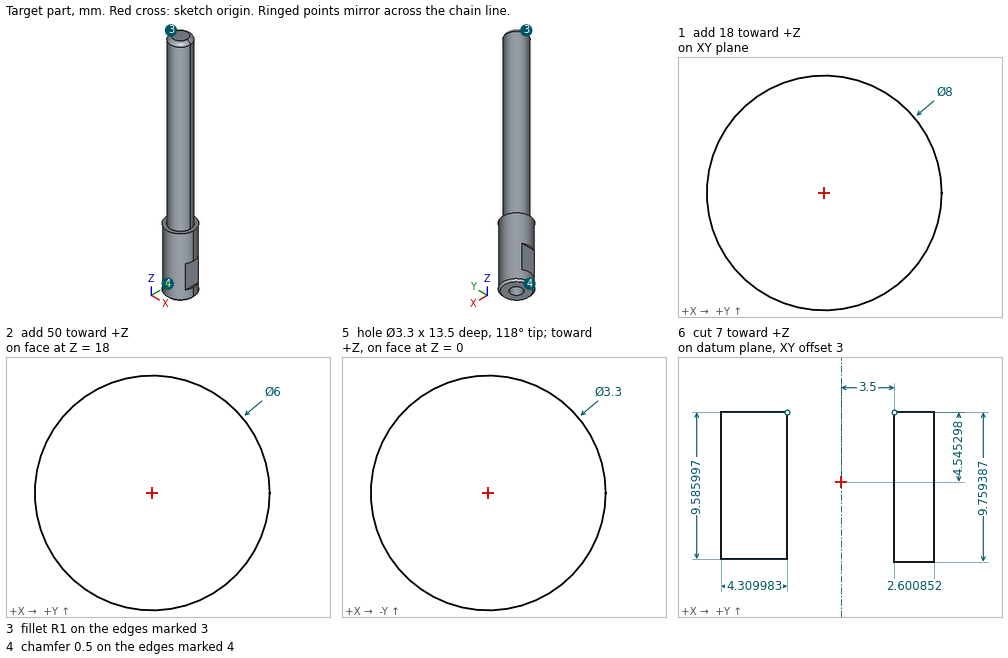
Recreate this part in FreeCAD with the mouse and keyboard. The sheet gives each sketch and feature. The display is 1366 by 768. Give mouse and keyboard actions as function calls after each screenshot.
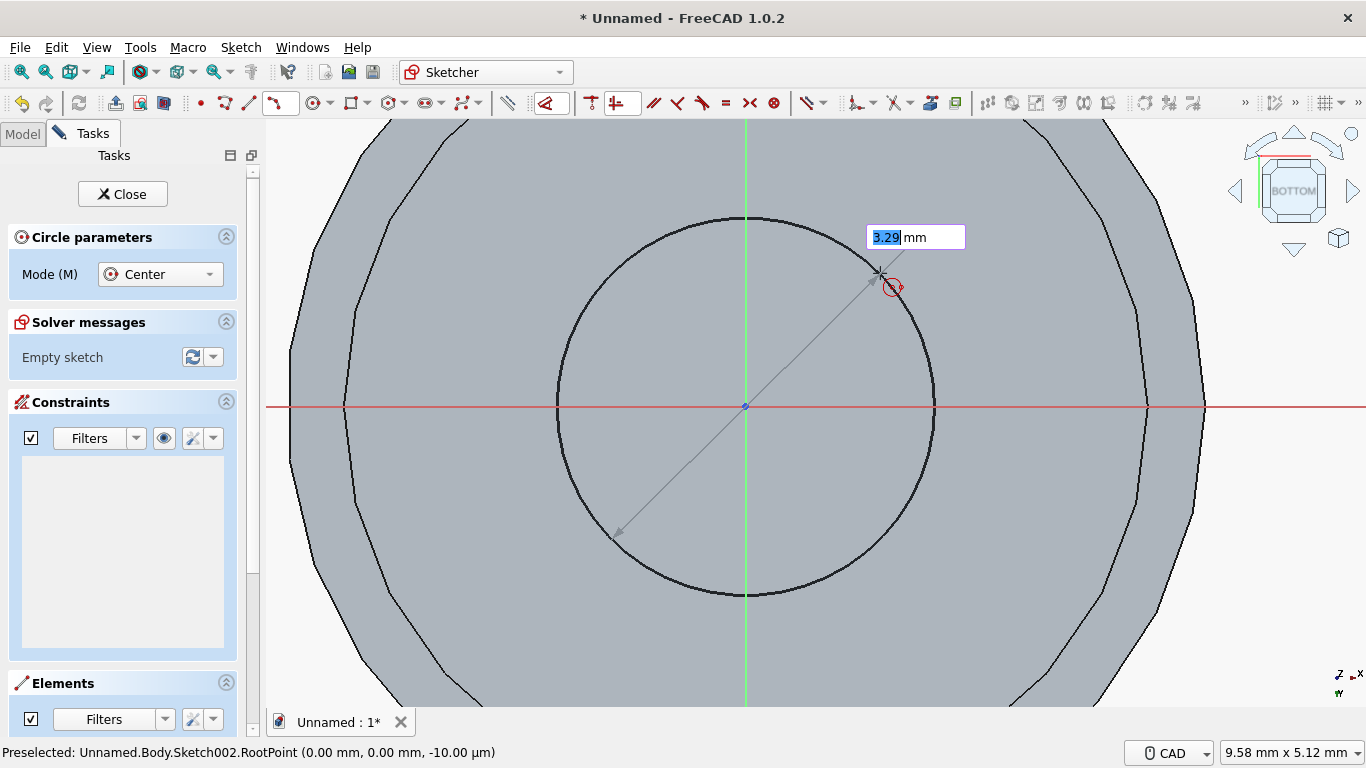
text(3.3)
key(Return)
key(Escape)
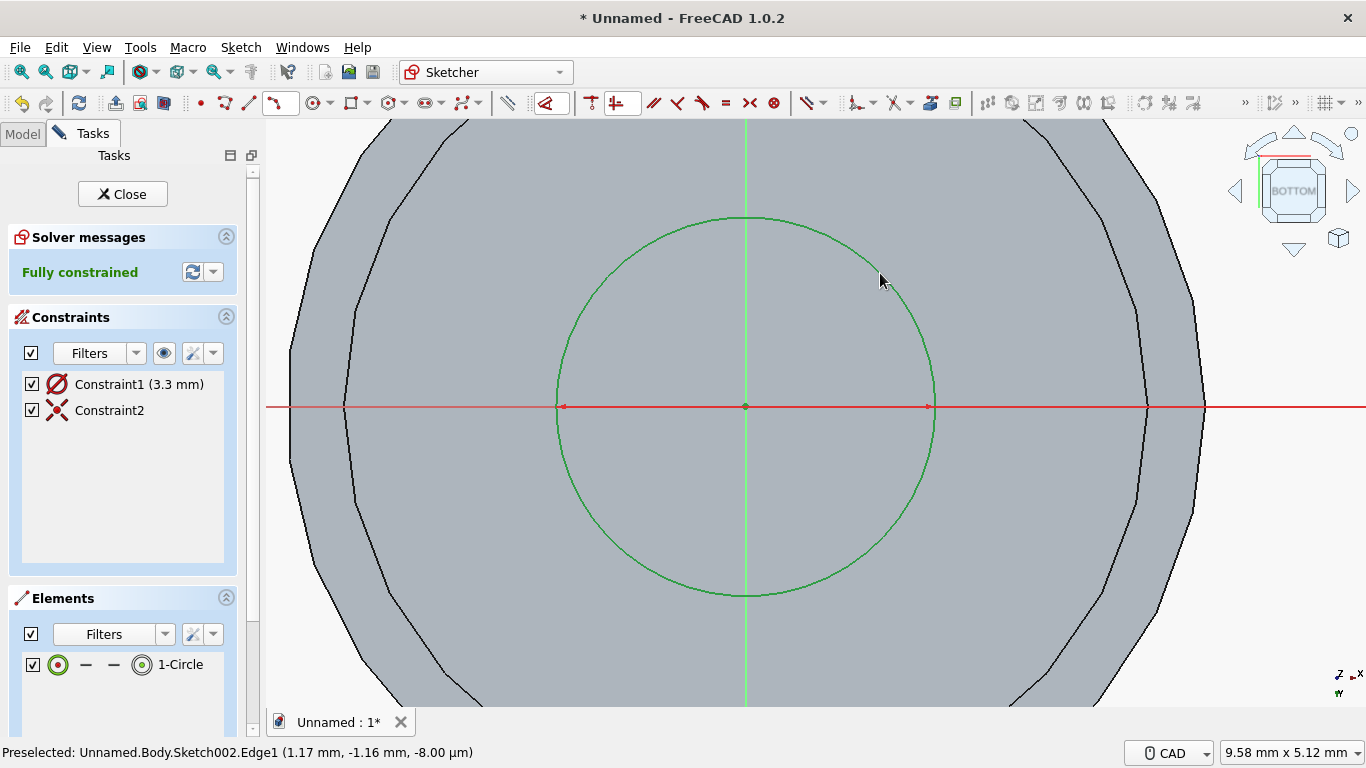
click(123, 194)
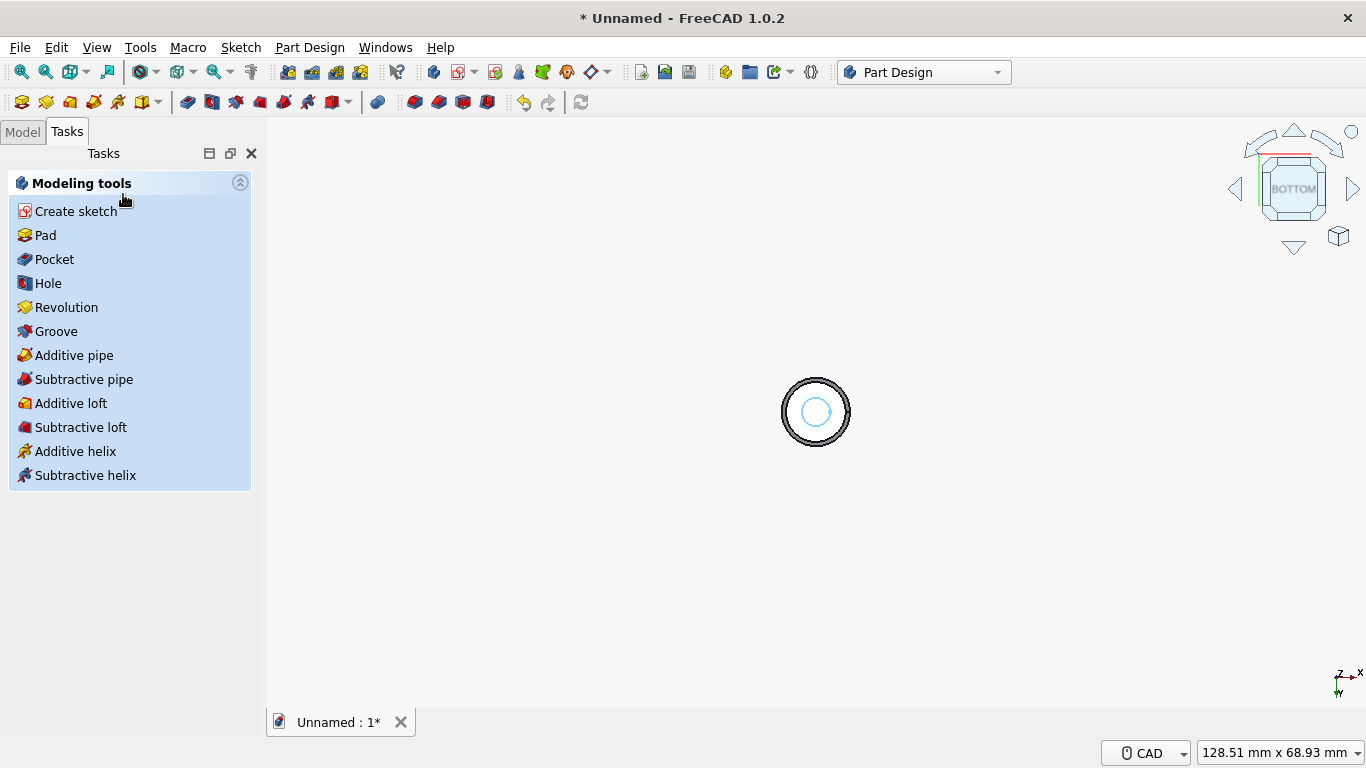
click(212, 102)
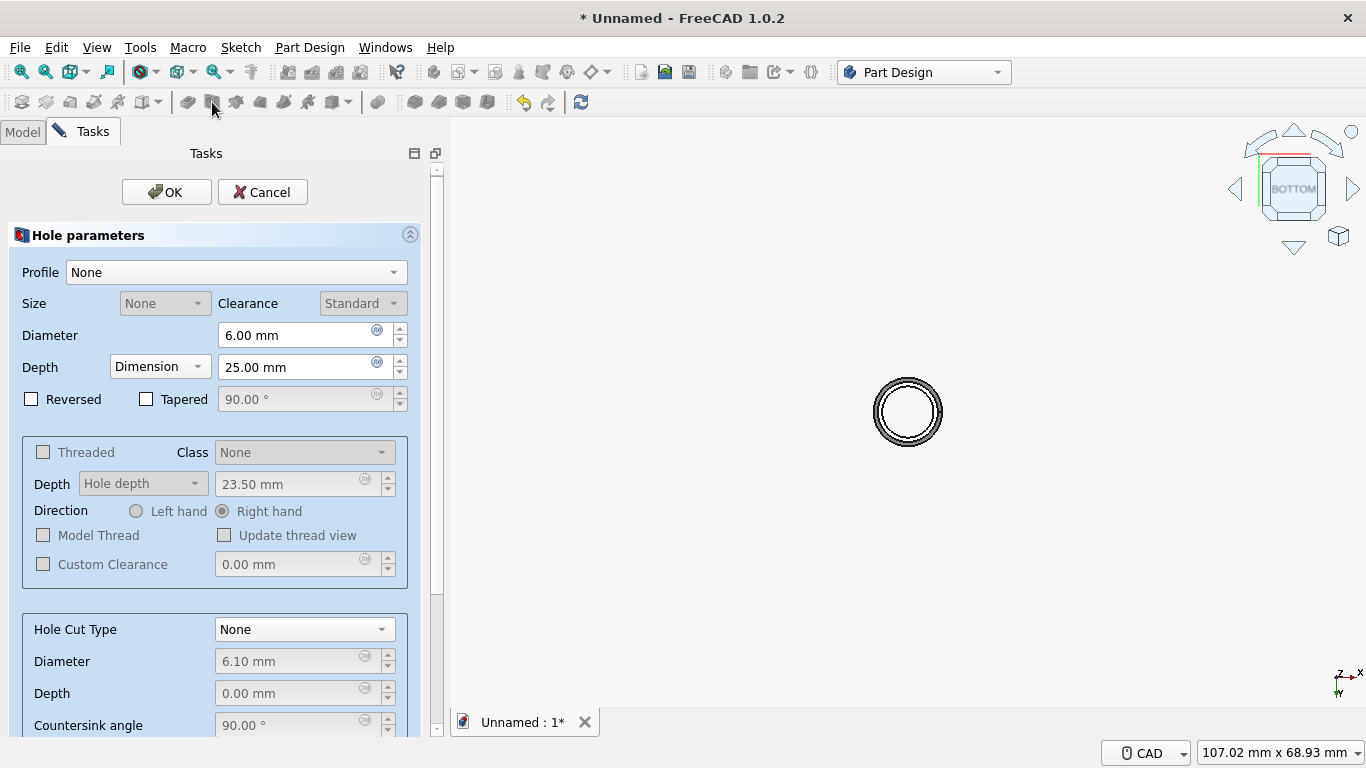
triple_click(305, 335)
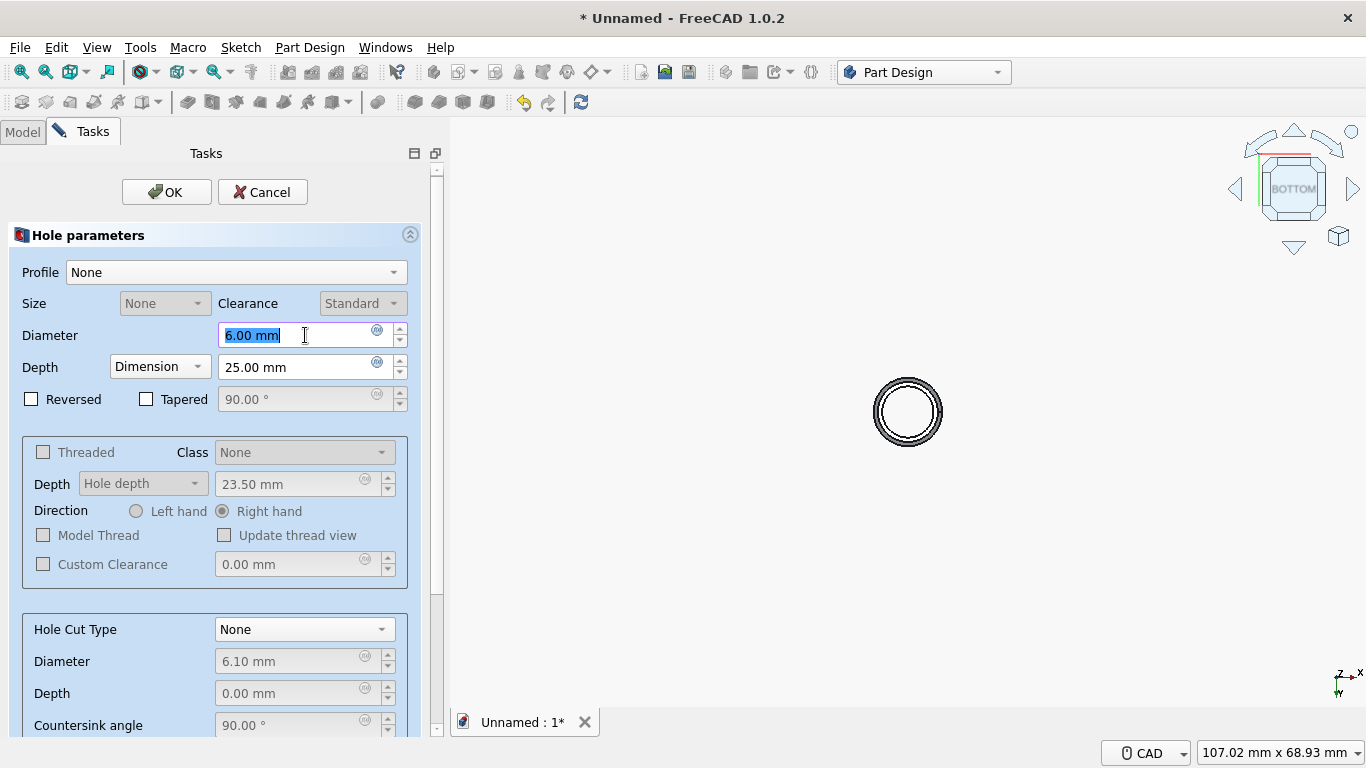
text(3.3)
key(Tab)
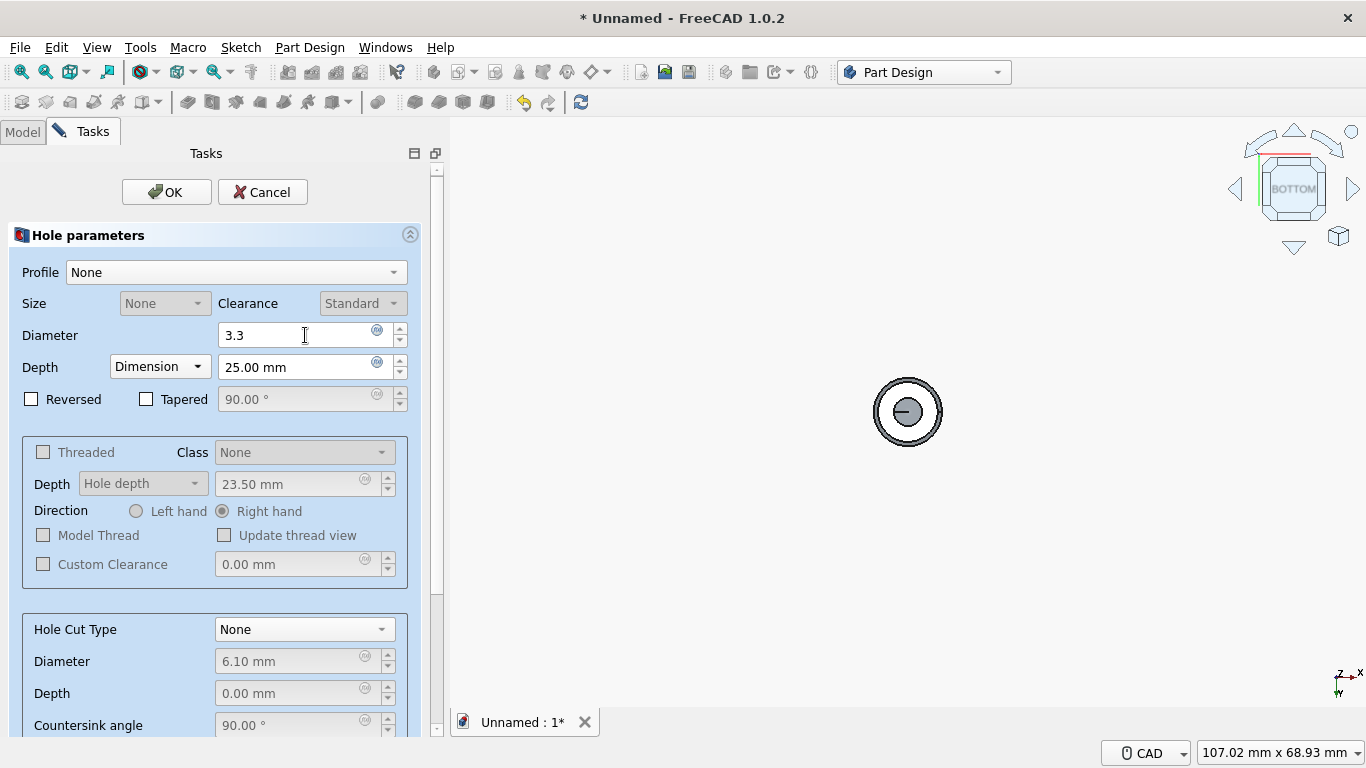
triple_click(305, 367)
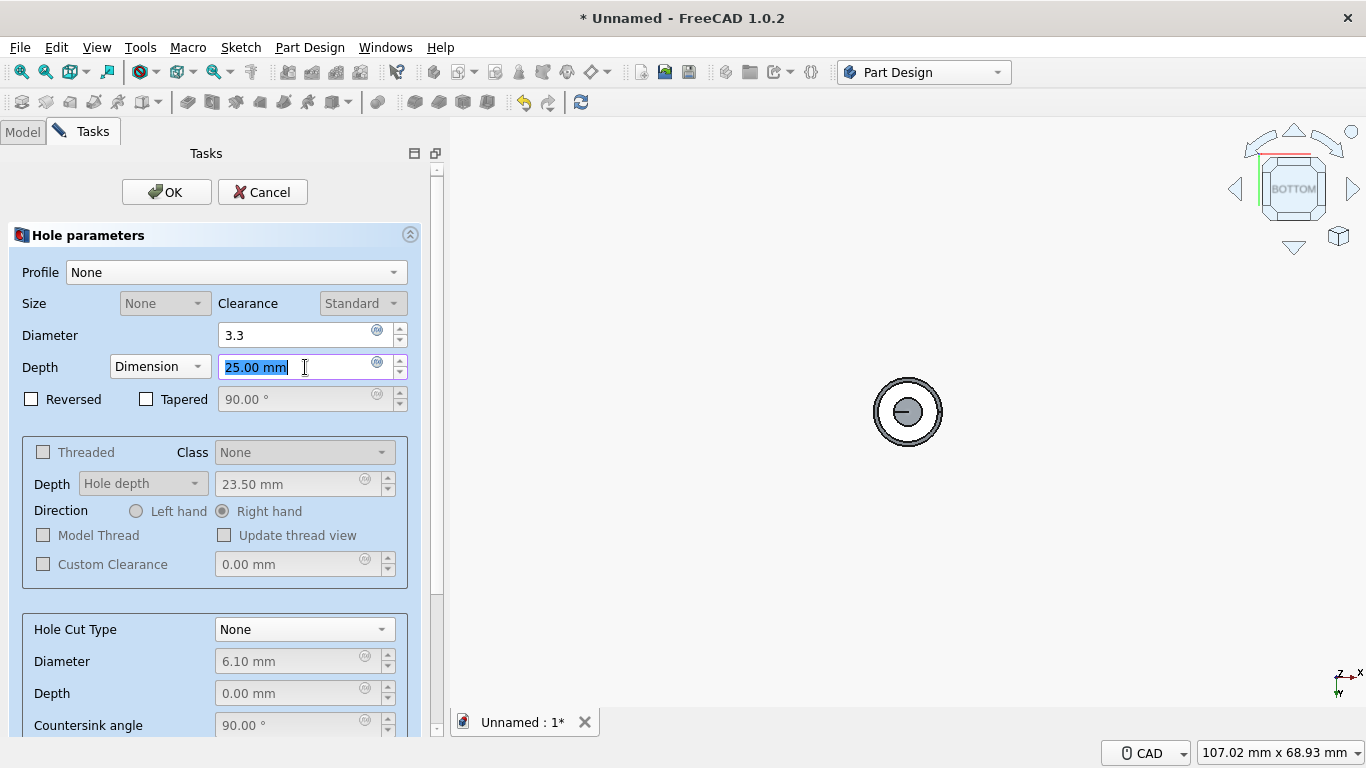
text(13.5)
key(Tab)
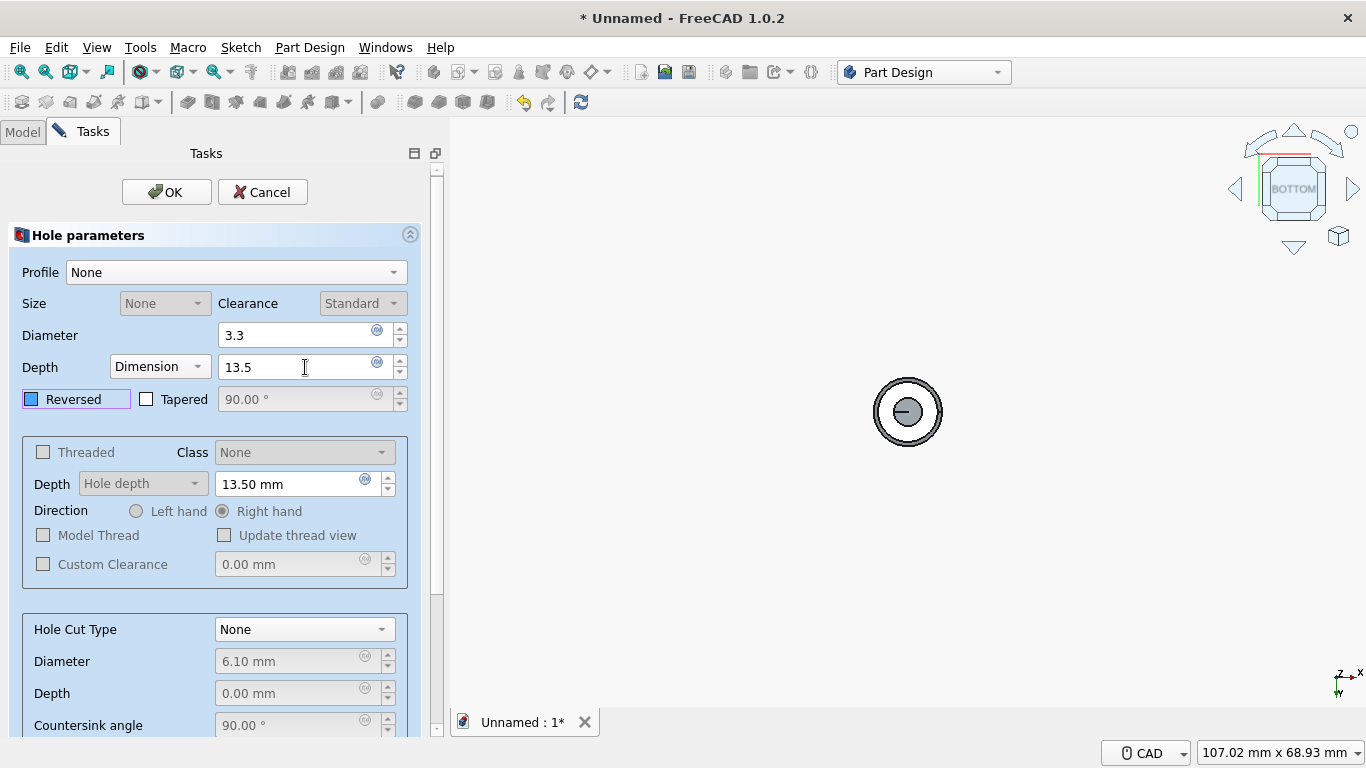
click(167, 192)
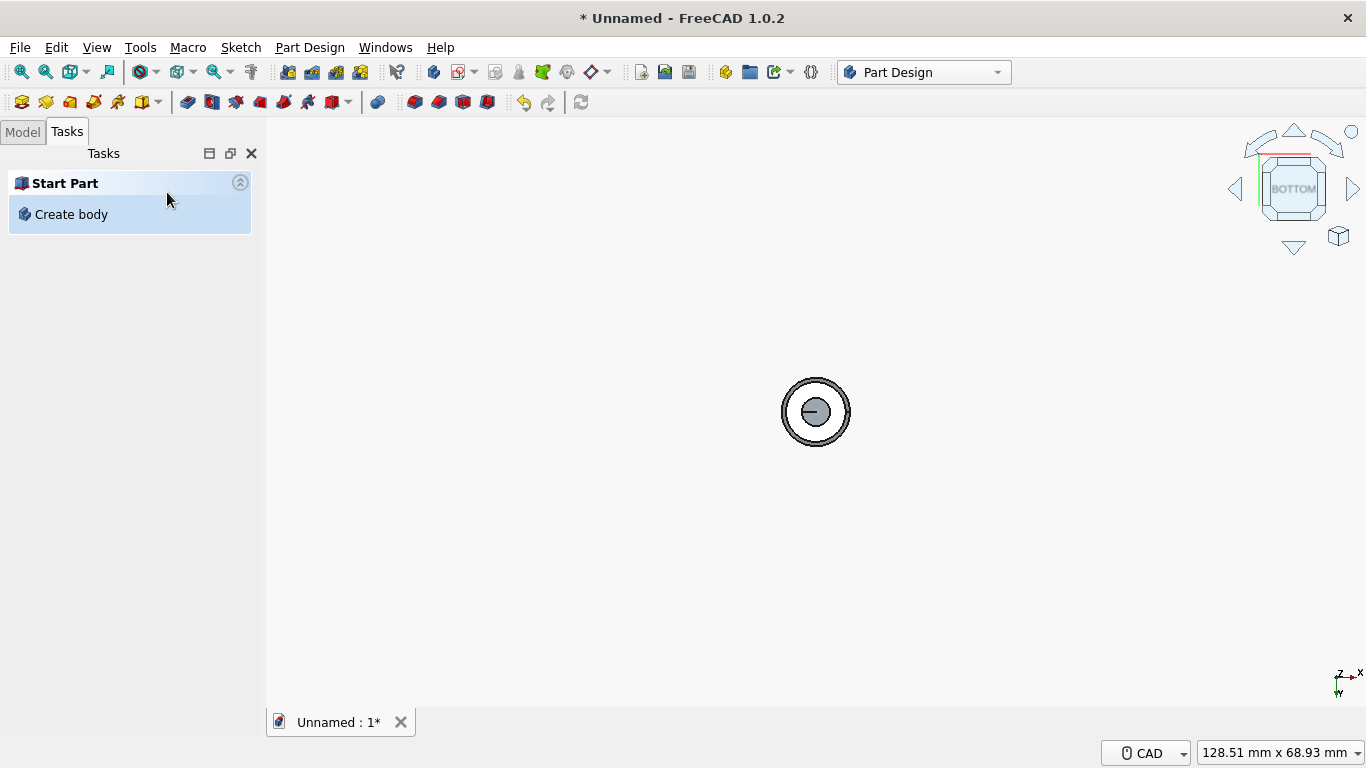
click(22, 72)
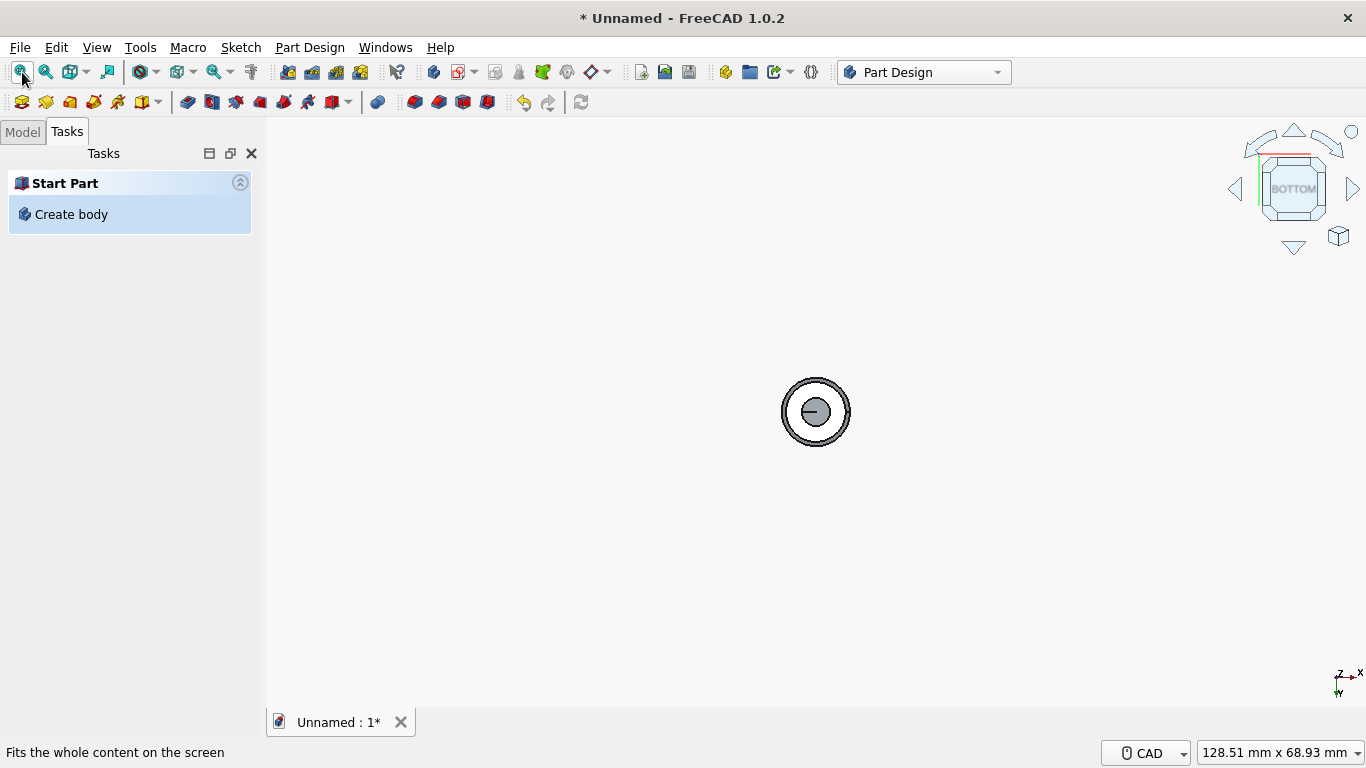
click(23, 131)